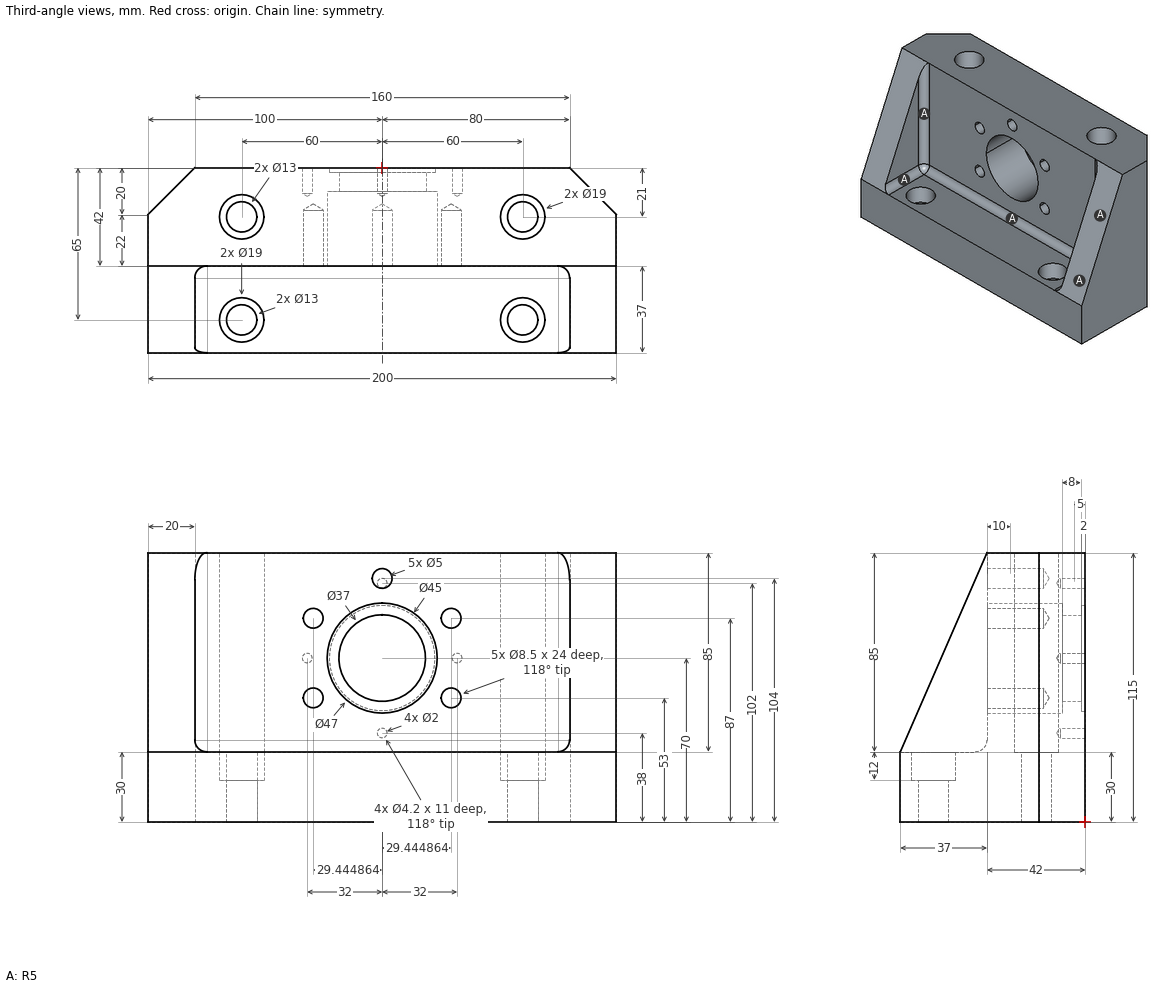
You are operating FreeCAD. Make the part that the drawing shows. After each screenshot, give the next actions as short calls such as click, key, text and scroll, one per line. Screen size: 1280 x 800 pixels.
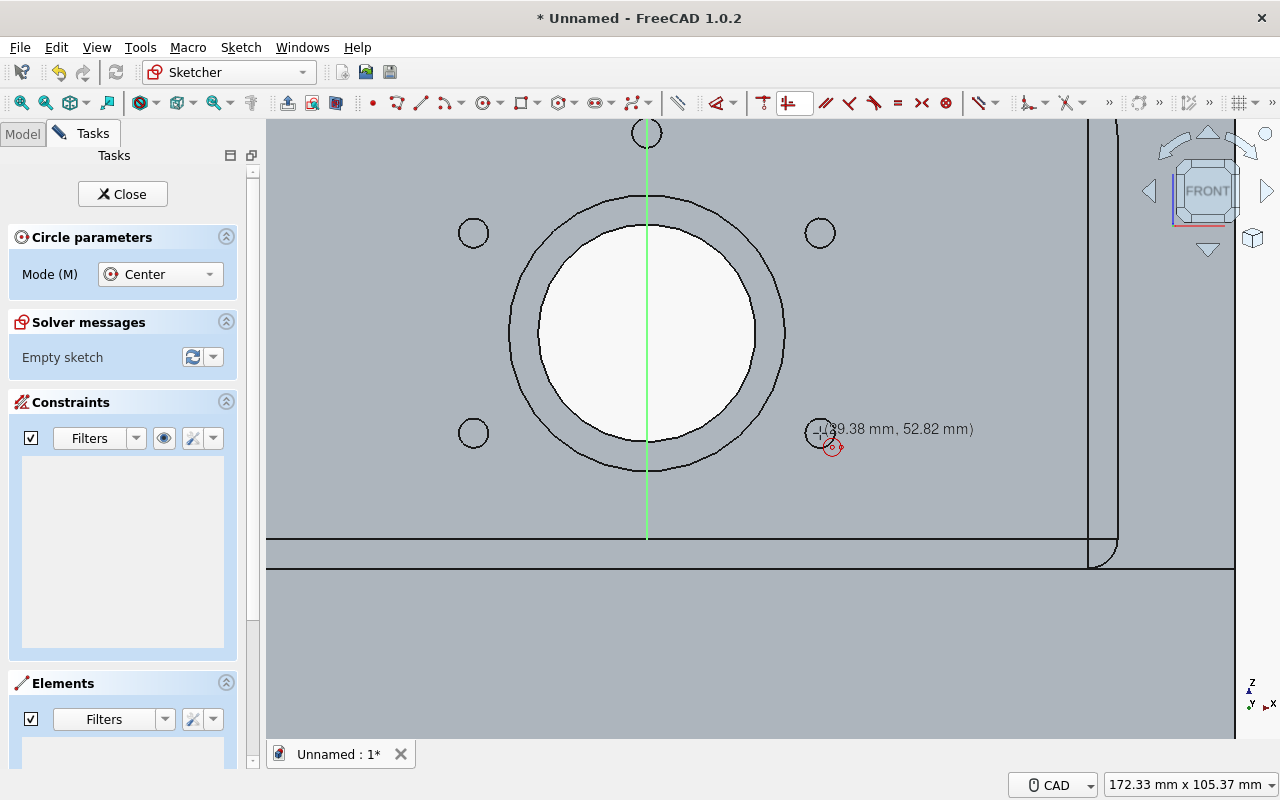
click(820, 433)
move(838, 415)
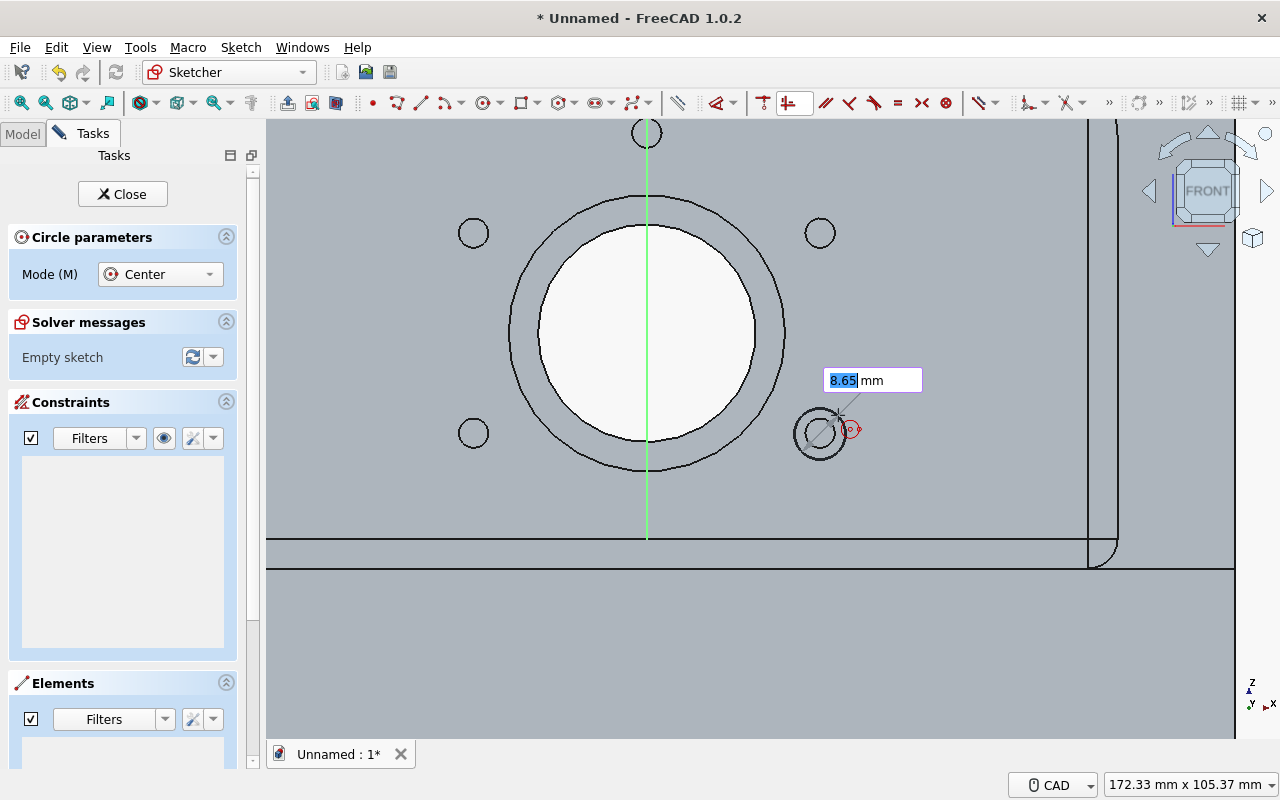
text(8.5)
key(Return)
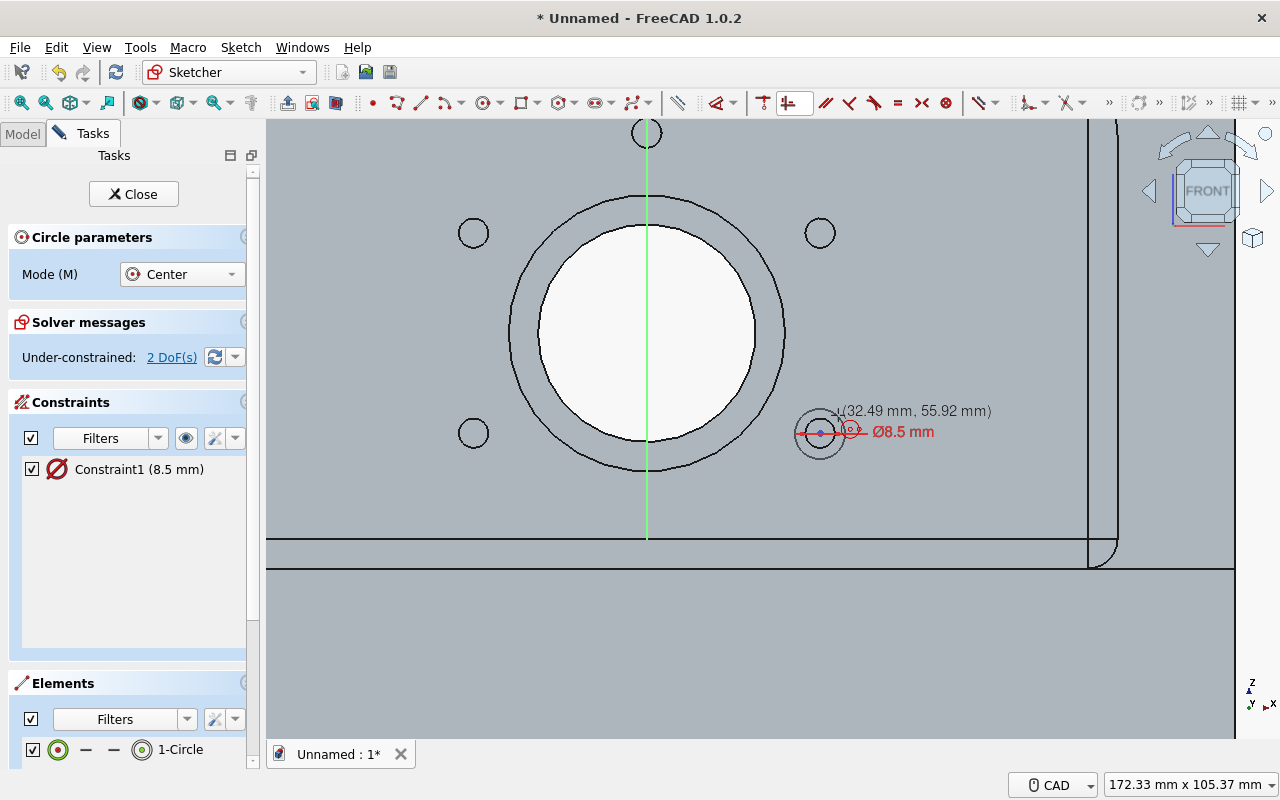
click(820, 233)
move(838, 215)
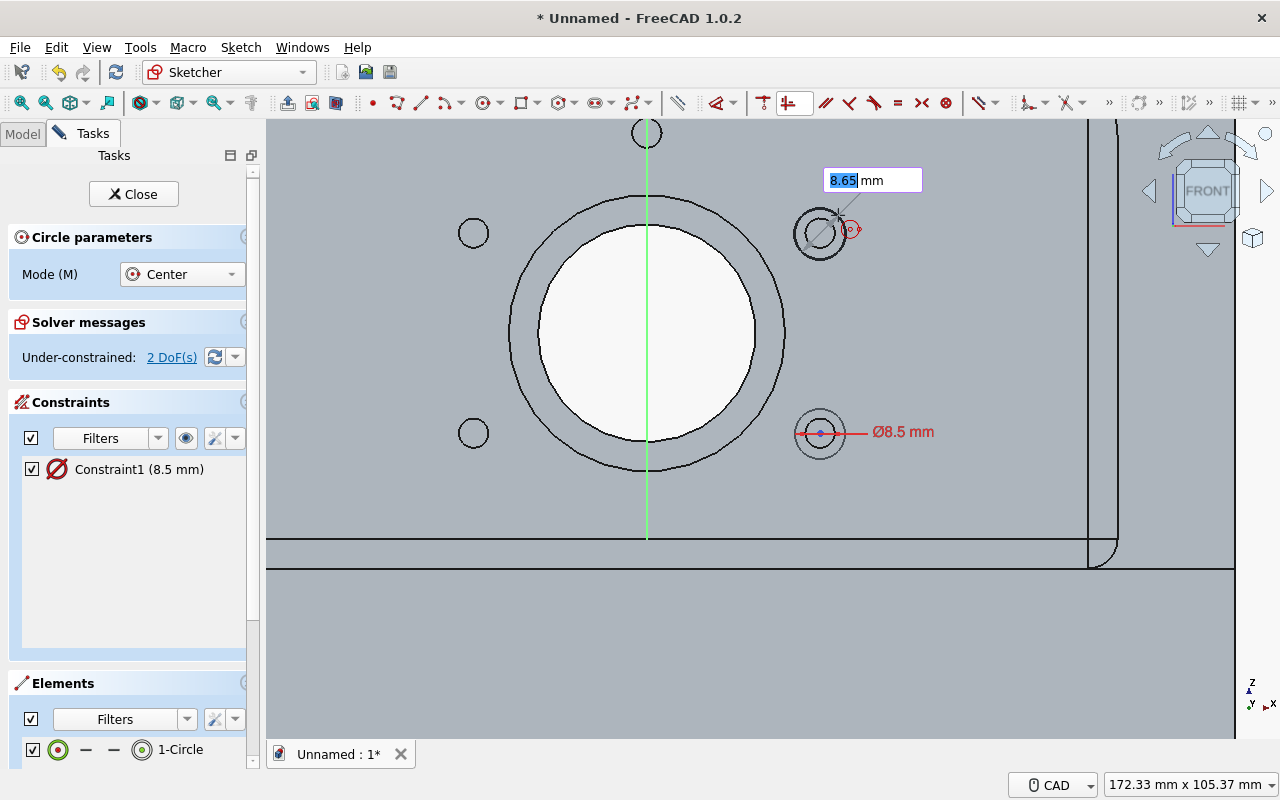
text(8.5)
key(Return)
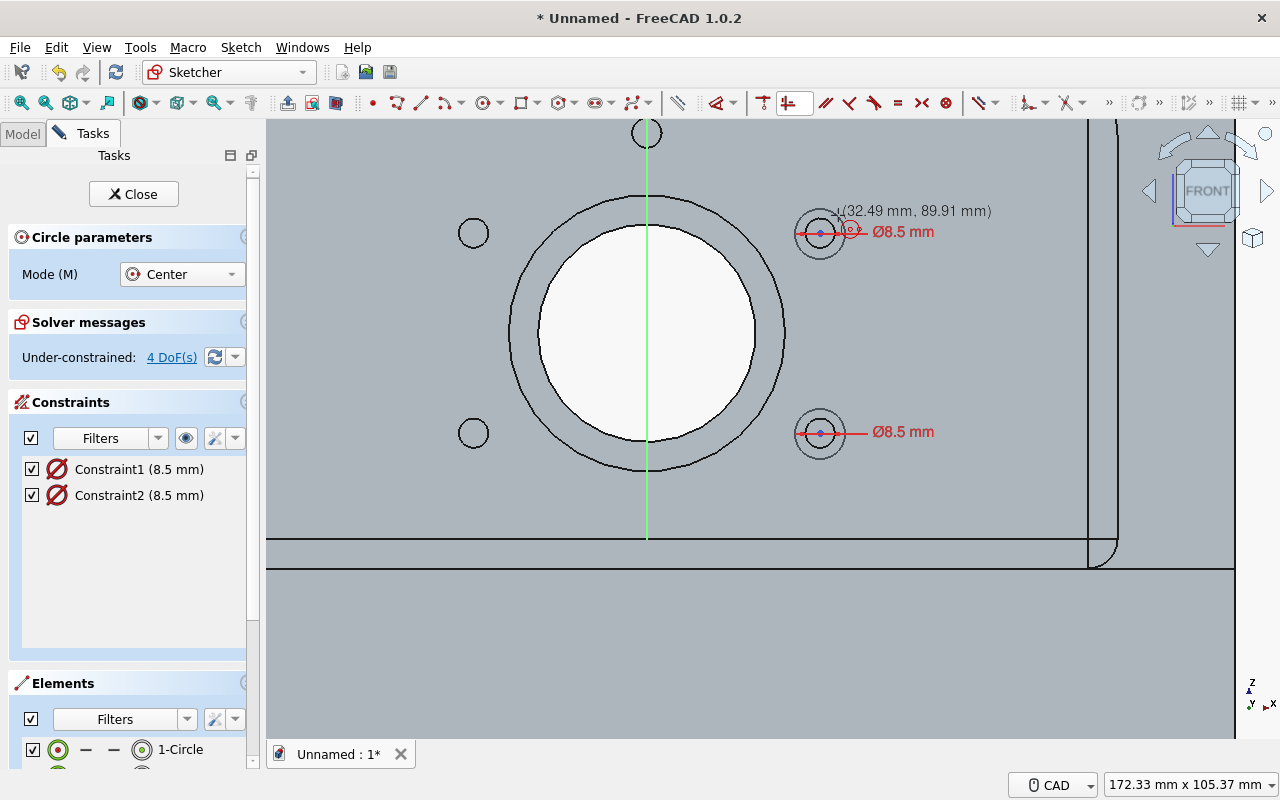
scroll(822, 434, down, 2)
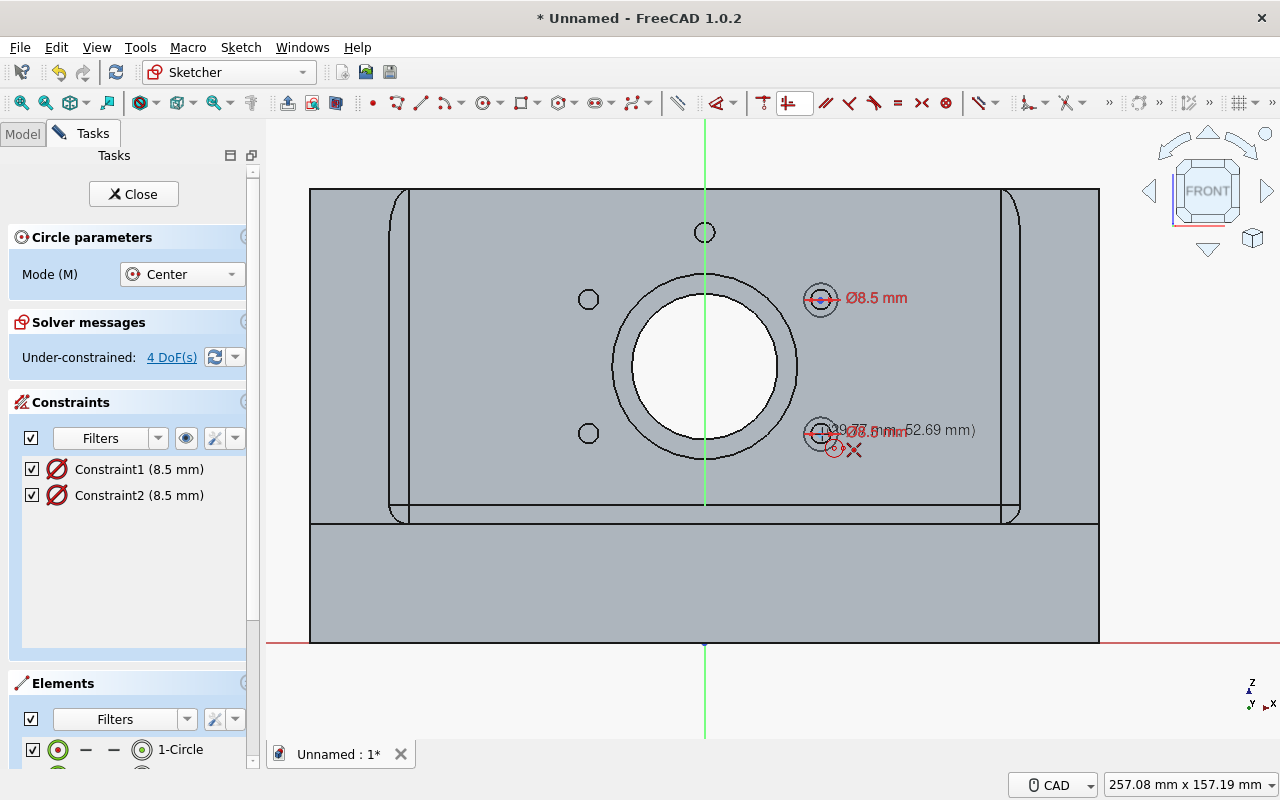
scroll(705, 232, up, 2)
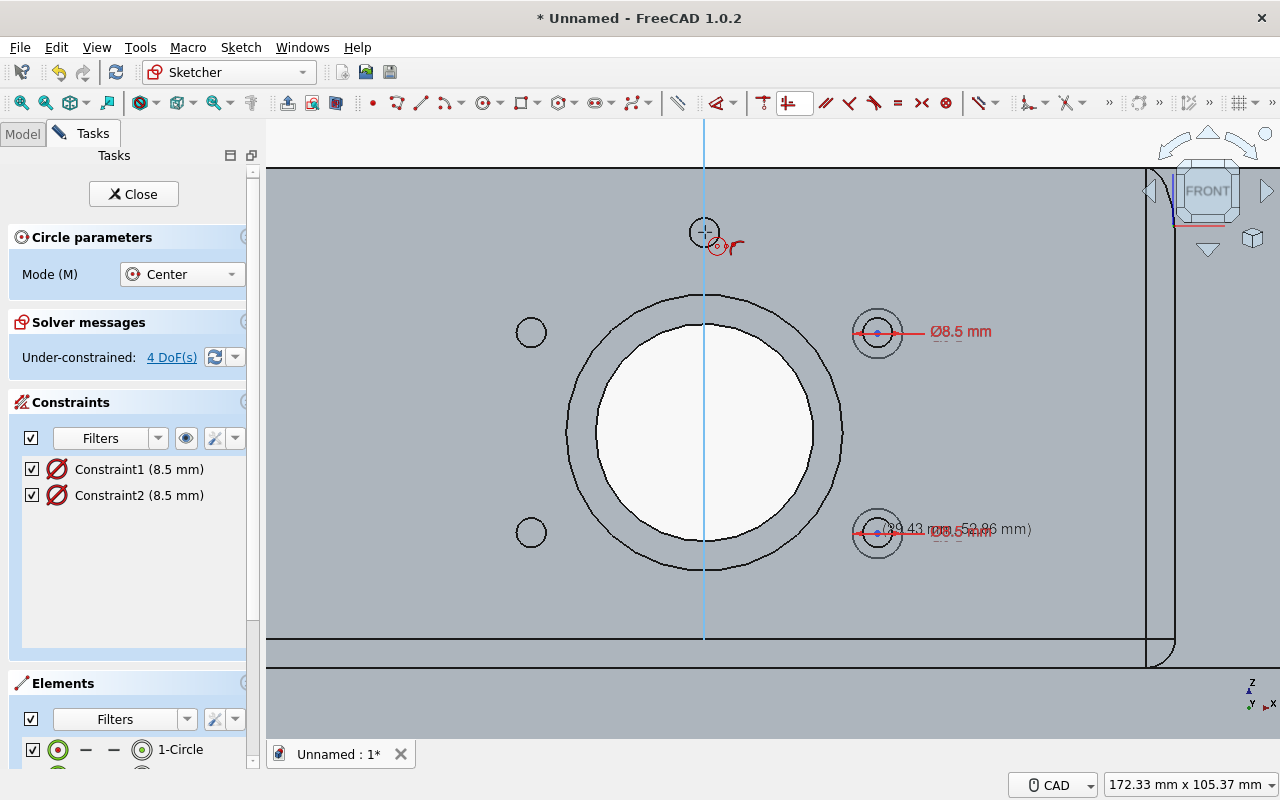
click(704, 233)
move(722, 215)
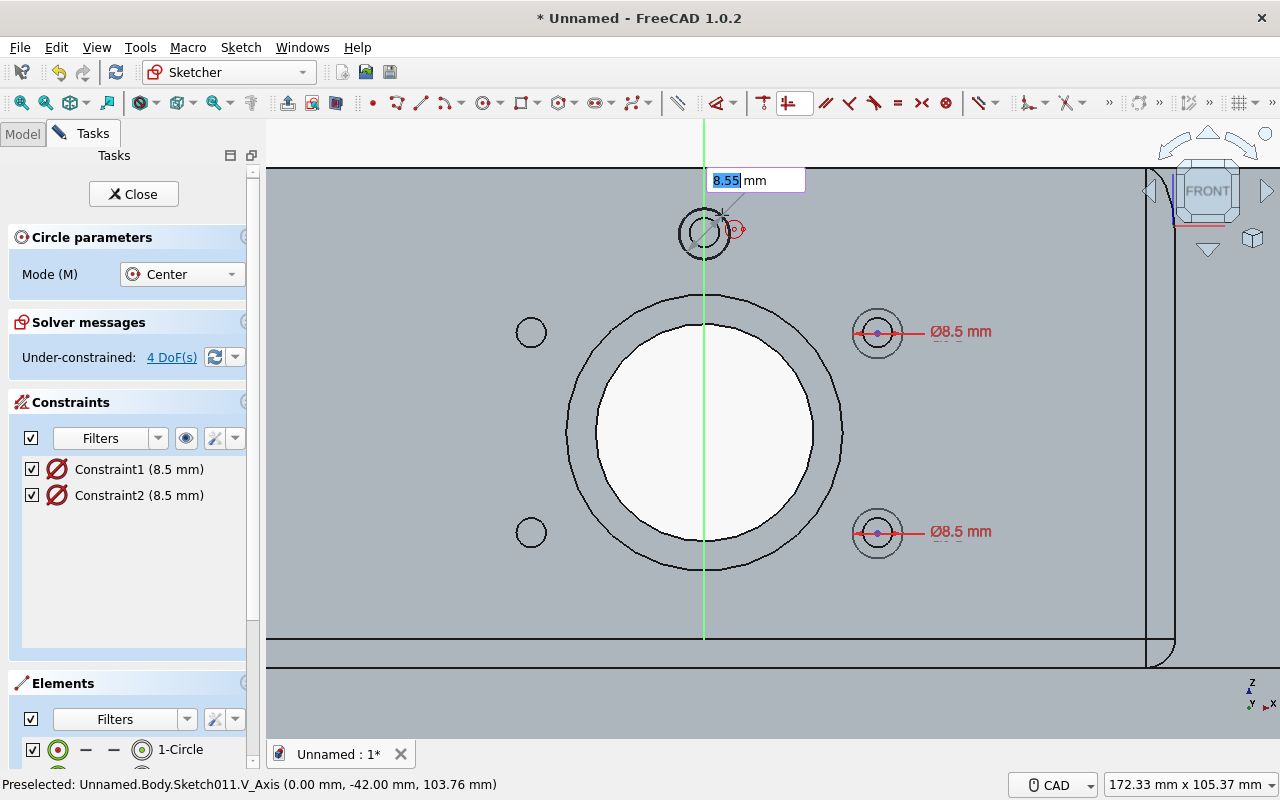
text(8.5)
key(Return)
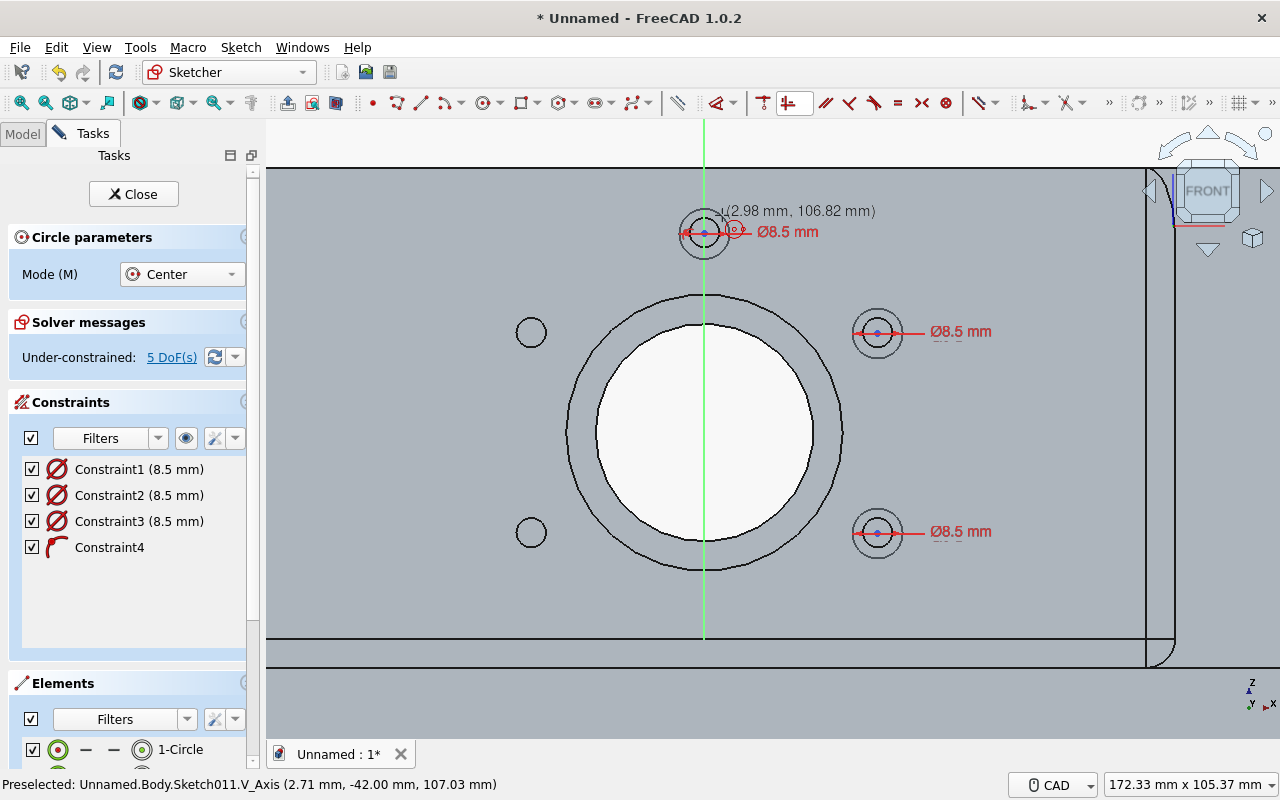
click(531, 333)
move(549, 315)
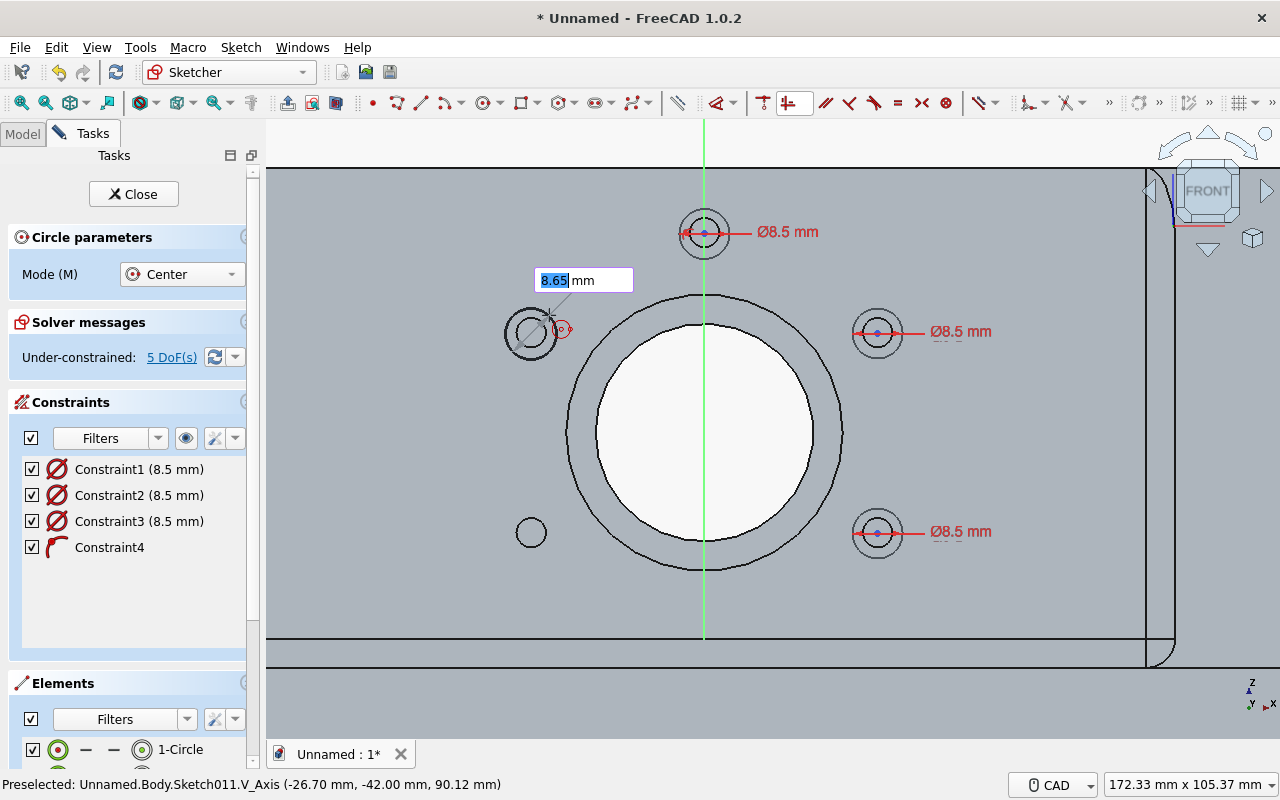
text(8.5)
key(Return)